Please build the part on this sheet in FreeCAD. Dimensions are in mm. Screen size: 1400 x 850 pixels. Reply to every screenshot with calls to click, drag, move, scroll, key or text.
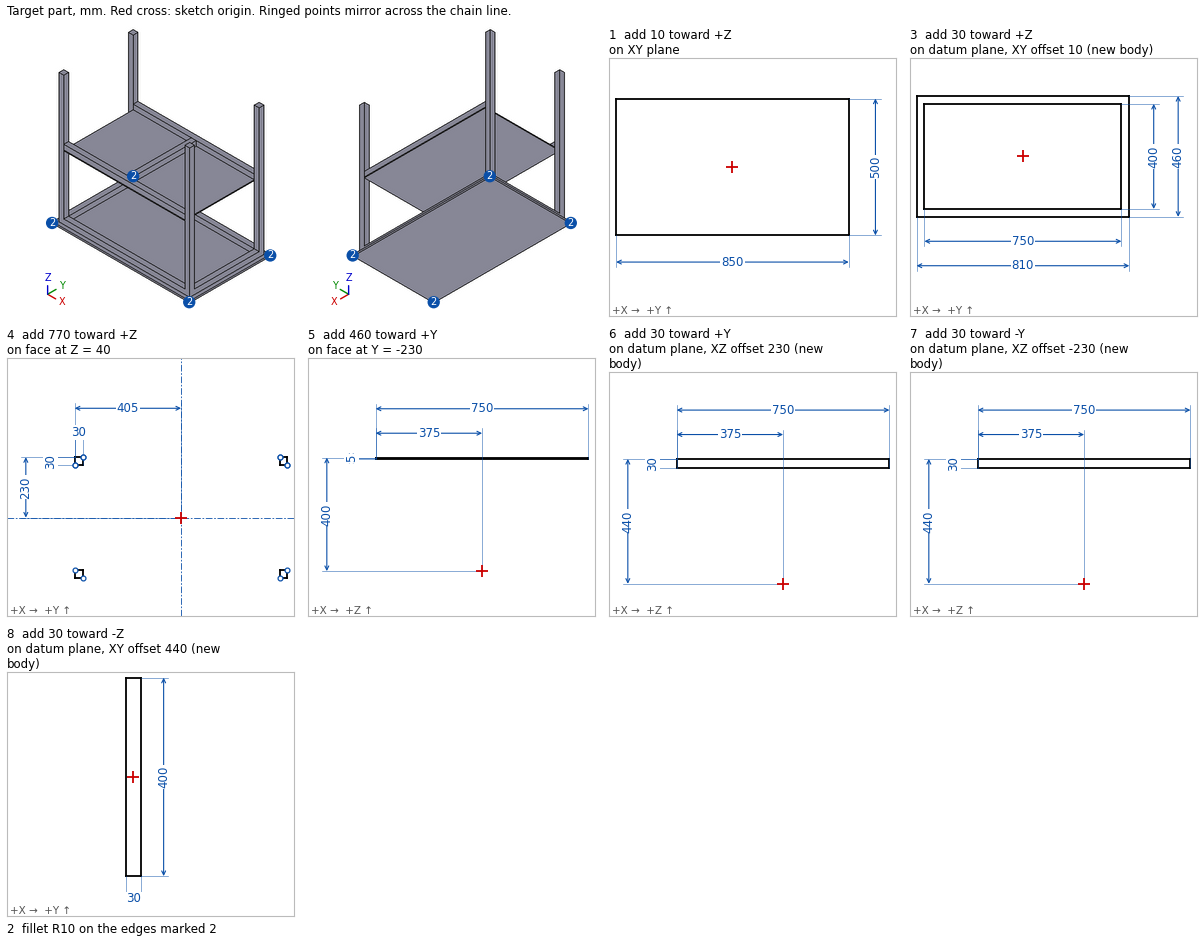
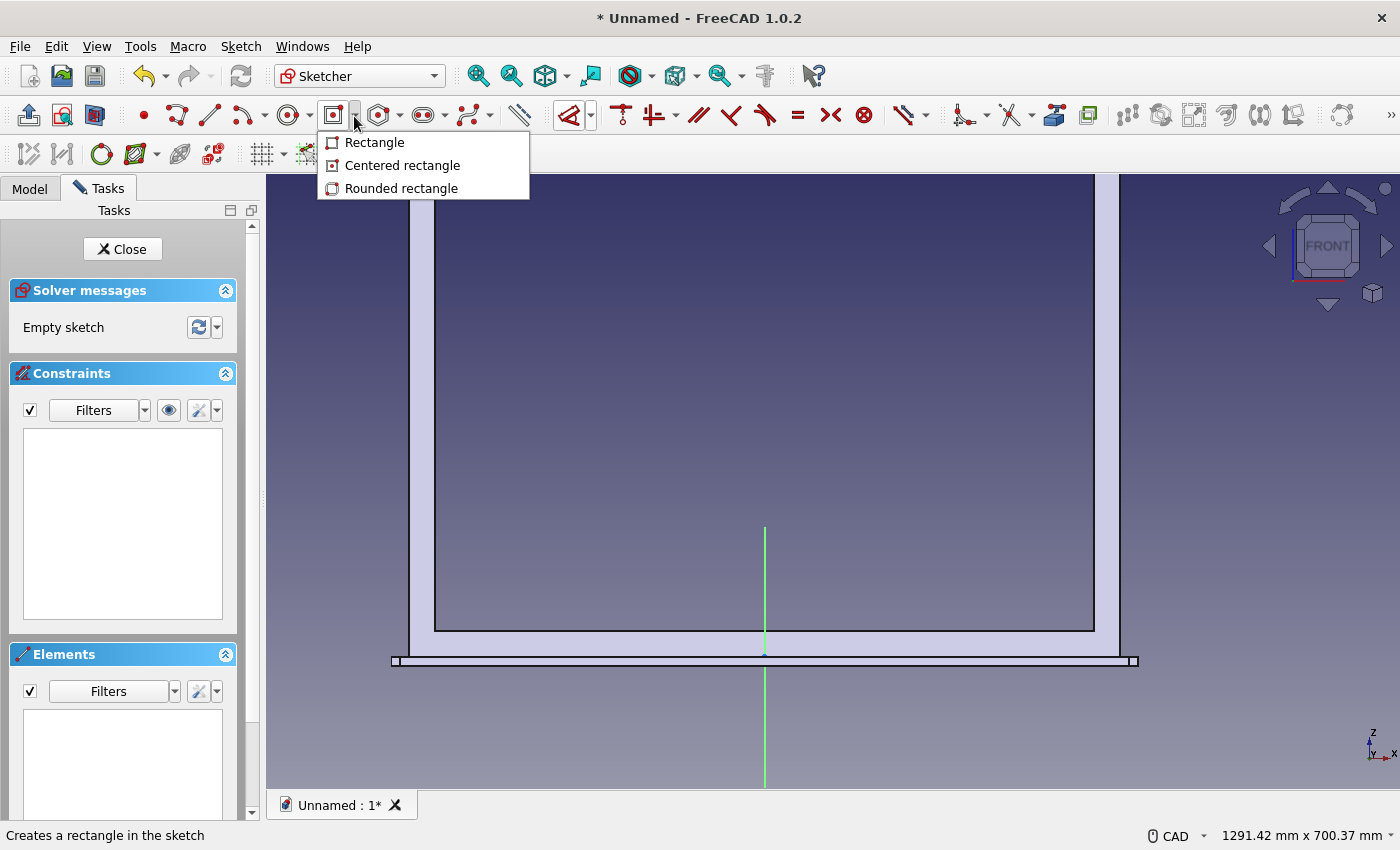
click(424, 142)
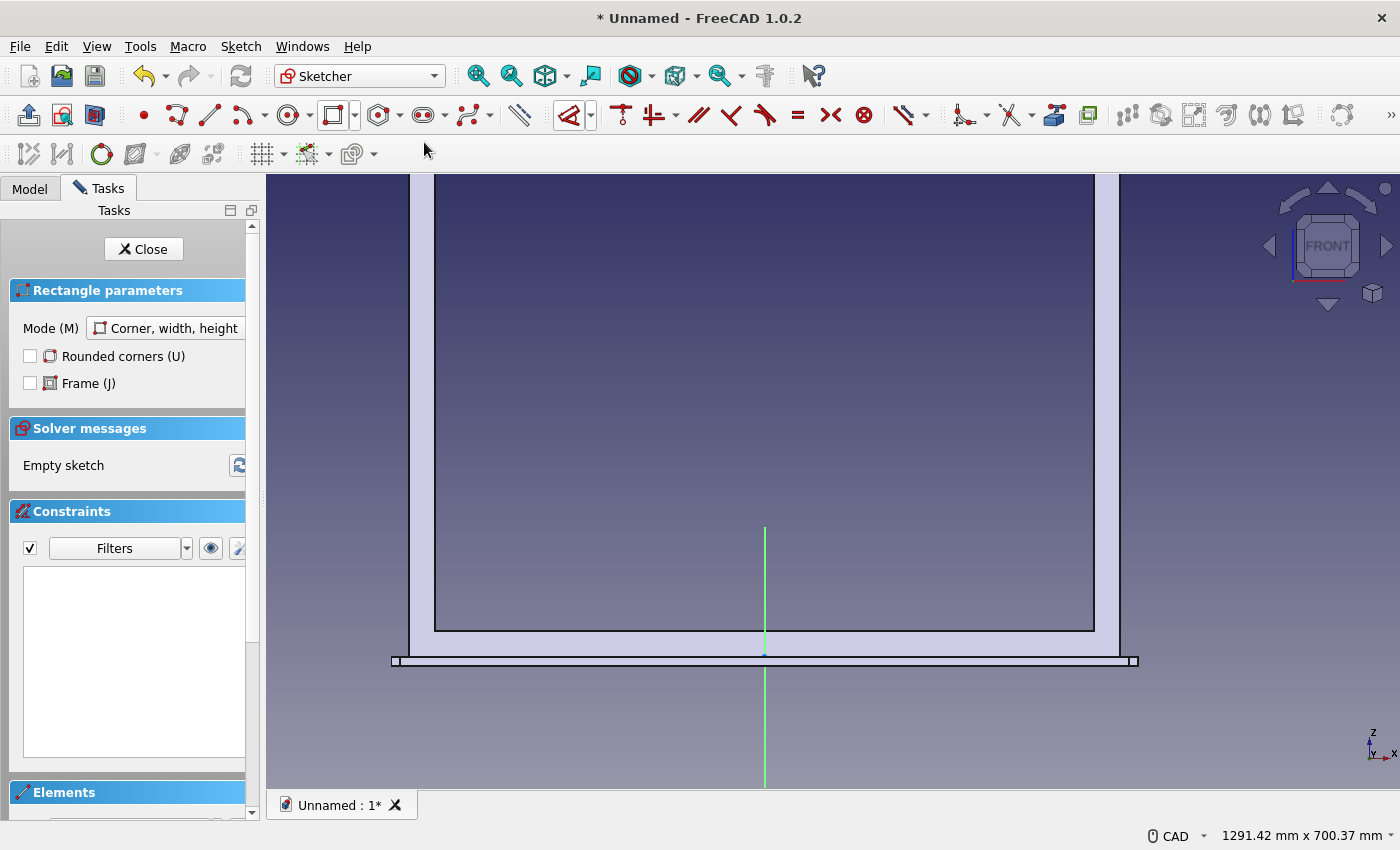
scroll(435, 306, up, 7)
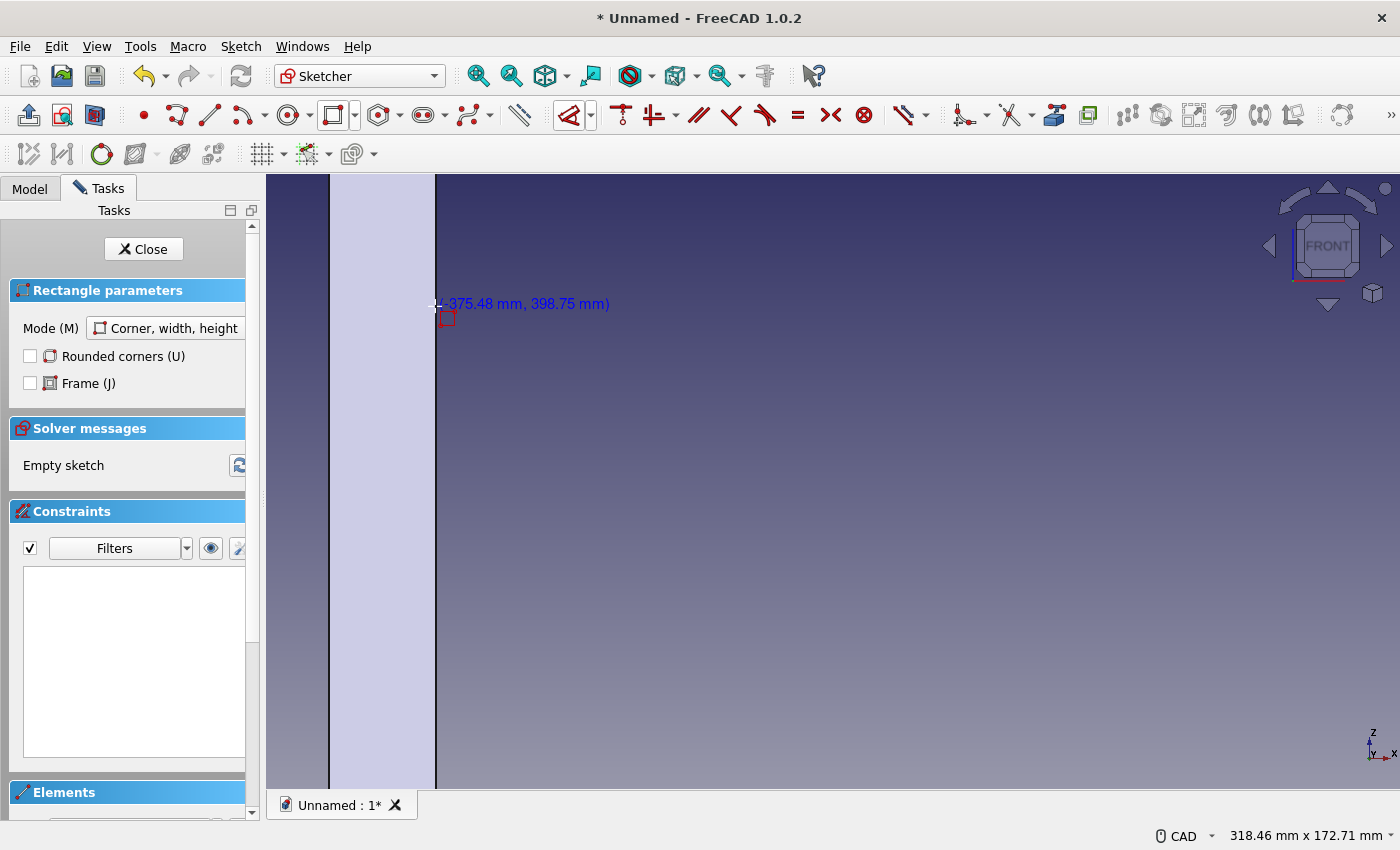
scroll(435, 306, down, 7)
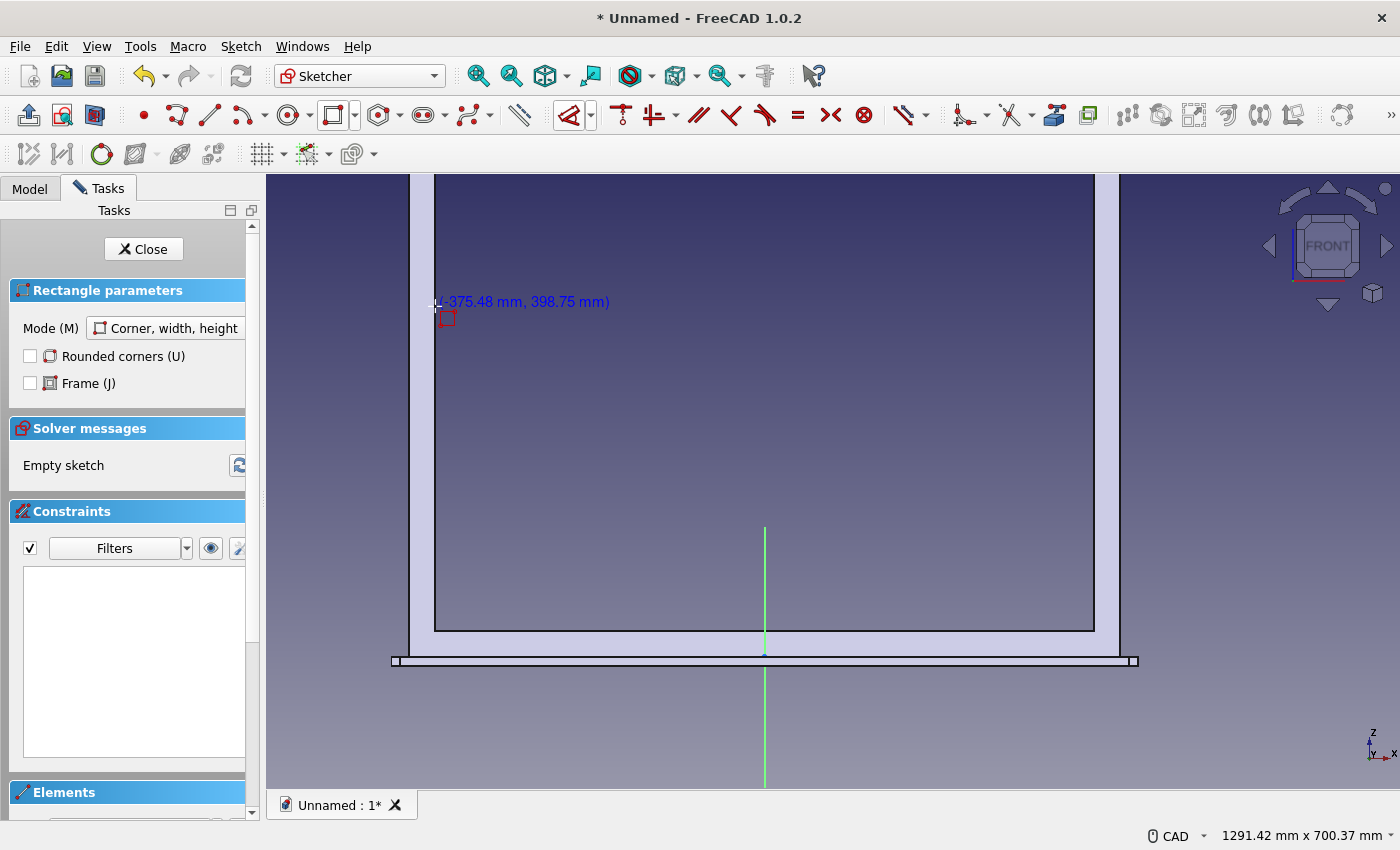
click(435, 306)
click(1094, 310)
key(Escape)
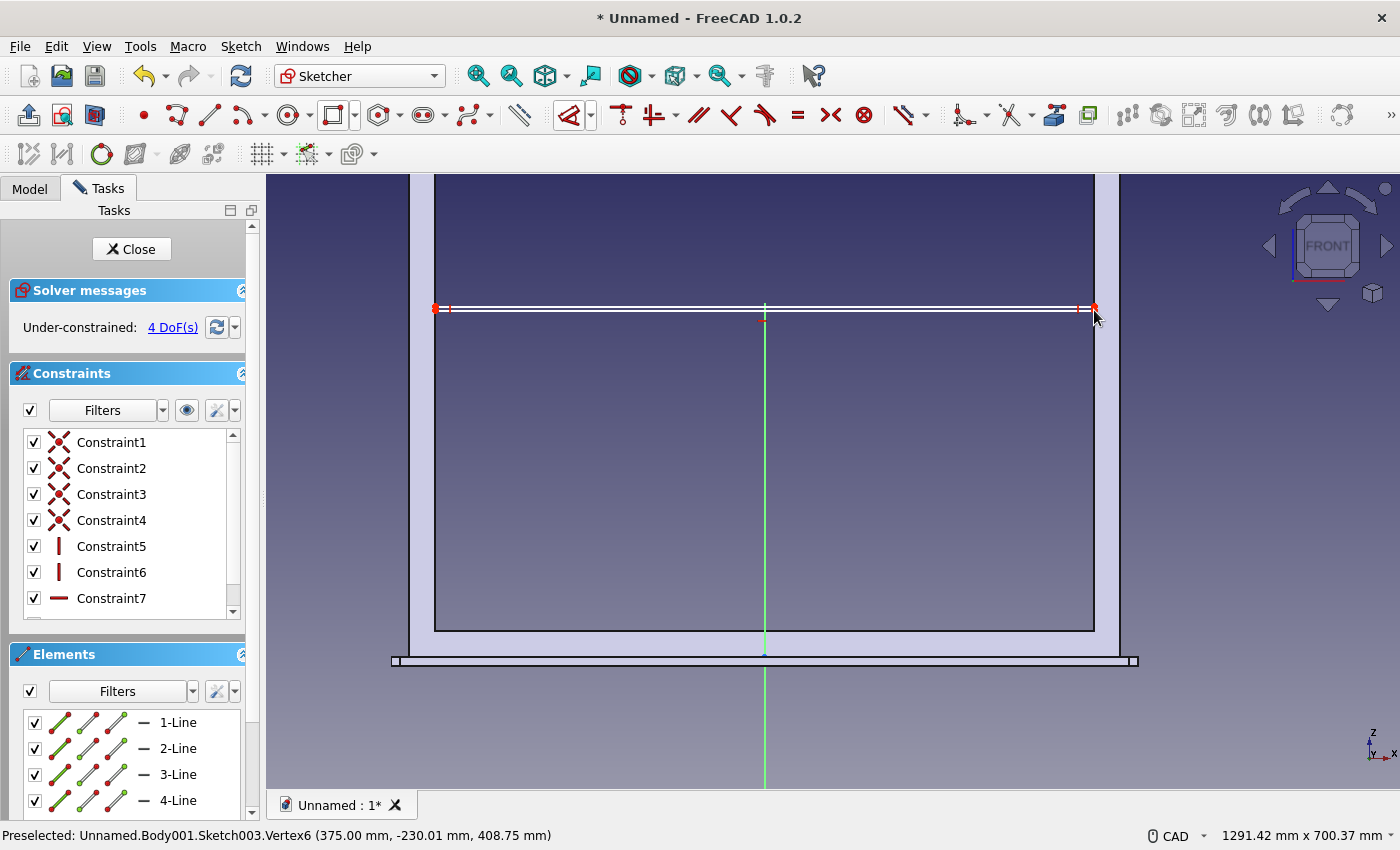
scroll(435, 309, up, 12)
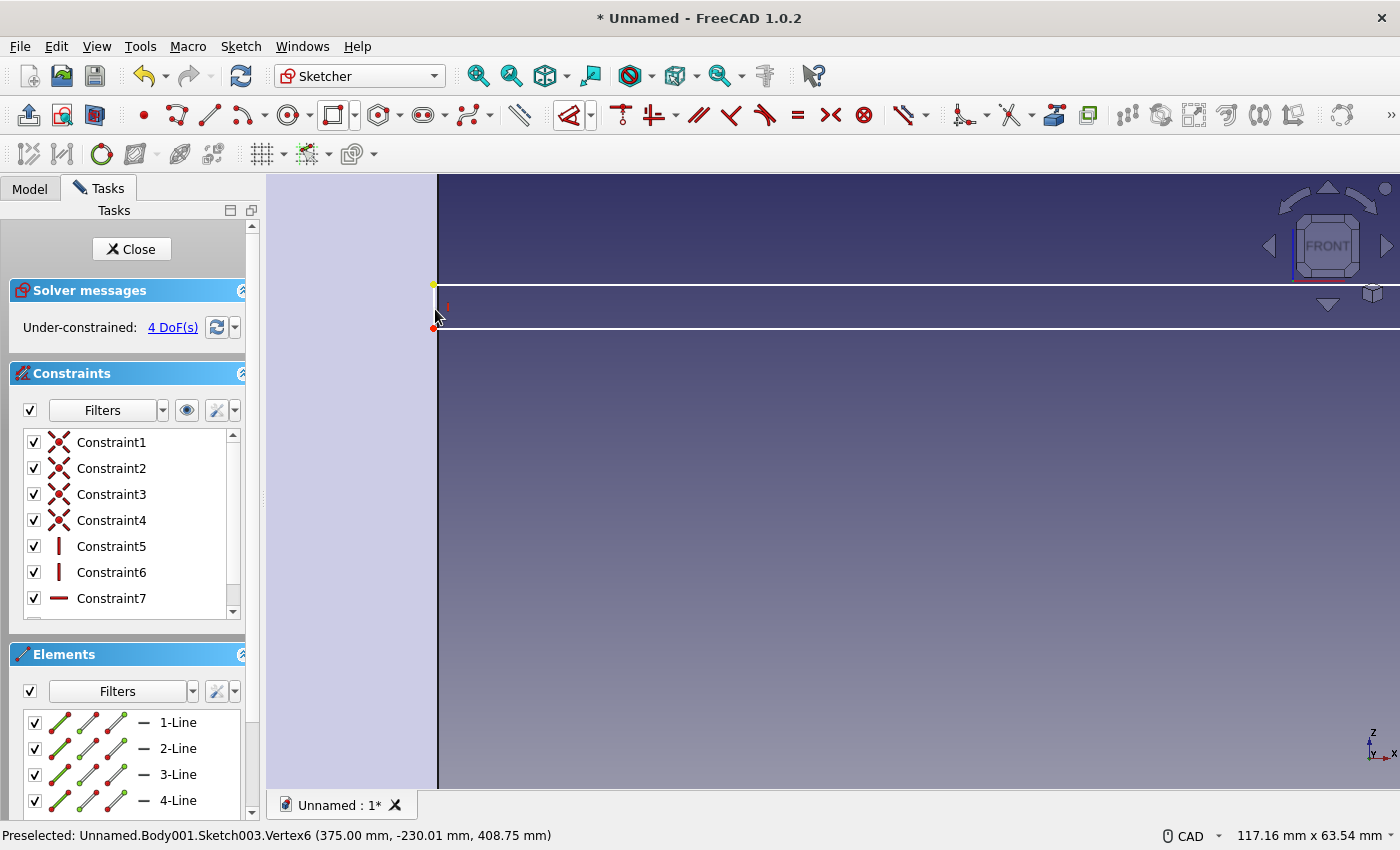
click(434, 307)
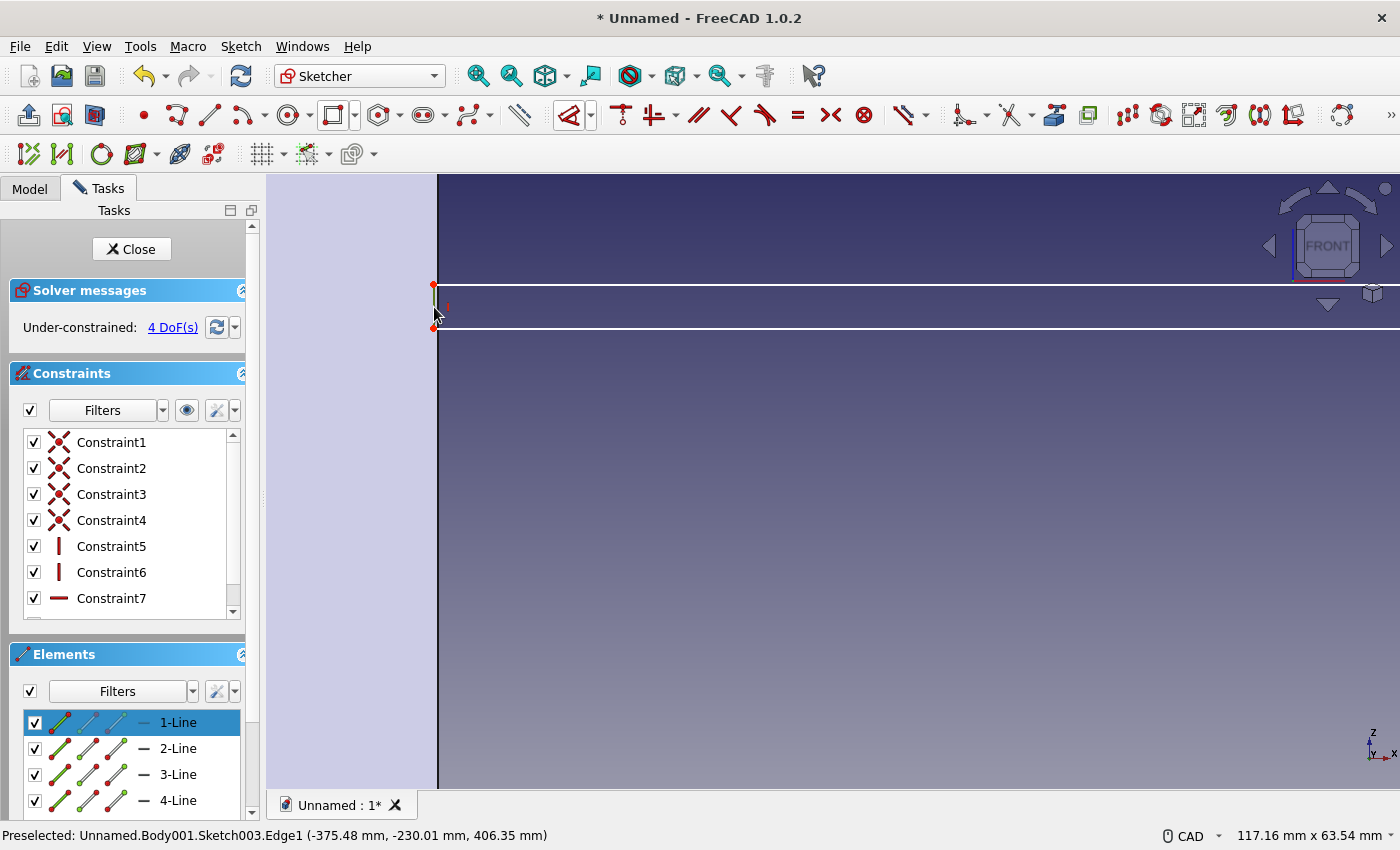
key(i)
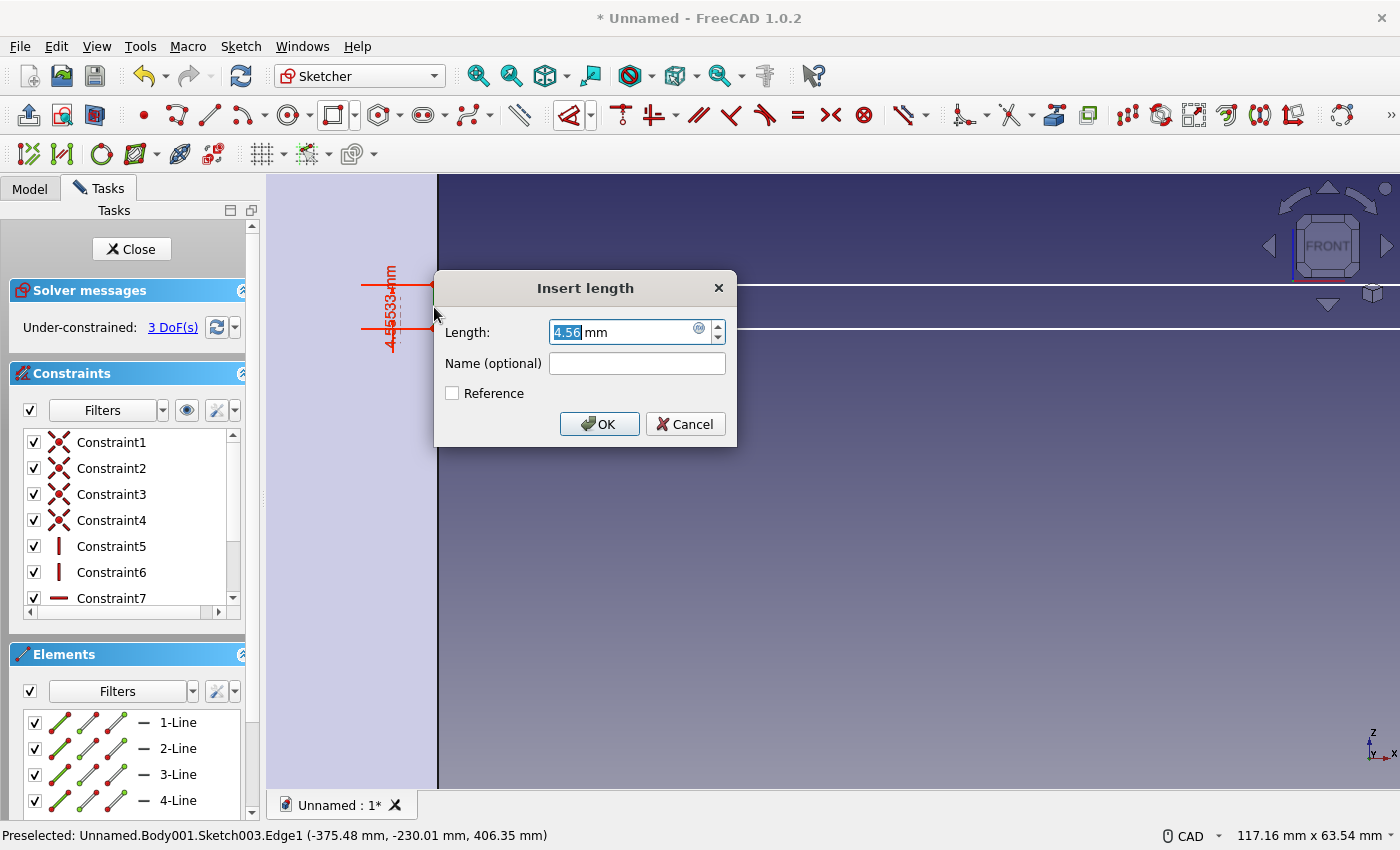
text(5)
key(Return)